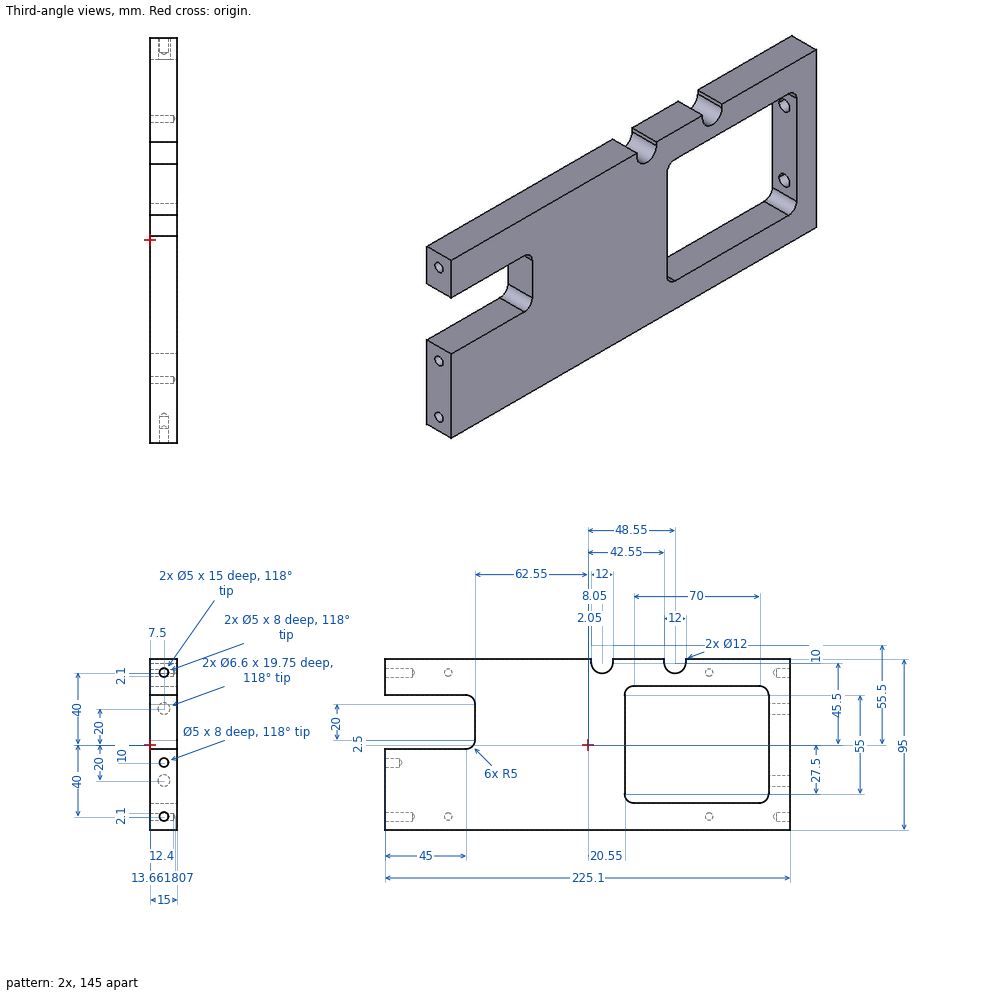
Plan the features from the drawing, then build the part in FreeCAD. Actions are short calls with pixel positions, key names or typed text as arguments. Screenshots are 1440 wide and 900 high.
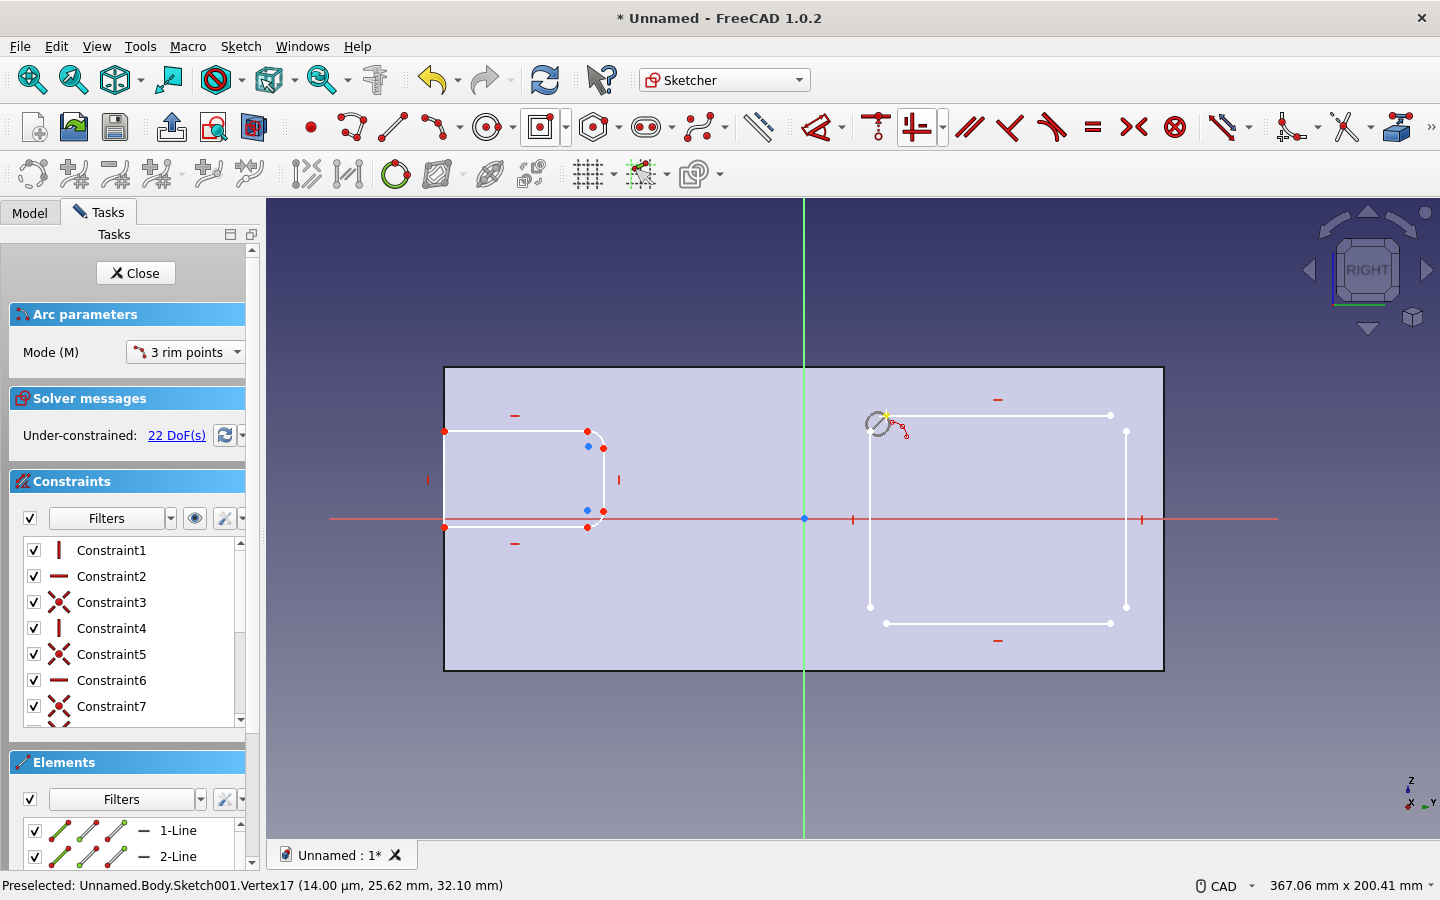
scroll(874, 419, up, 7)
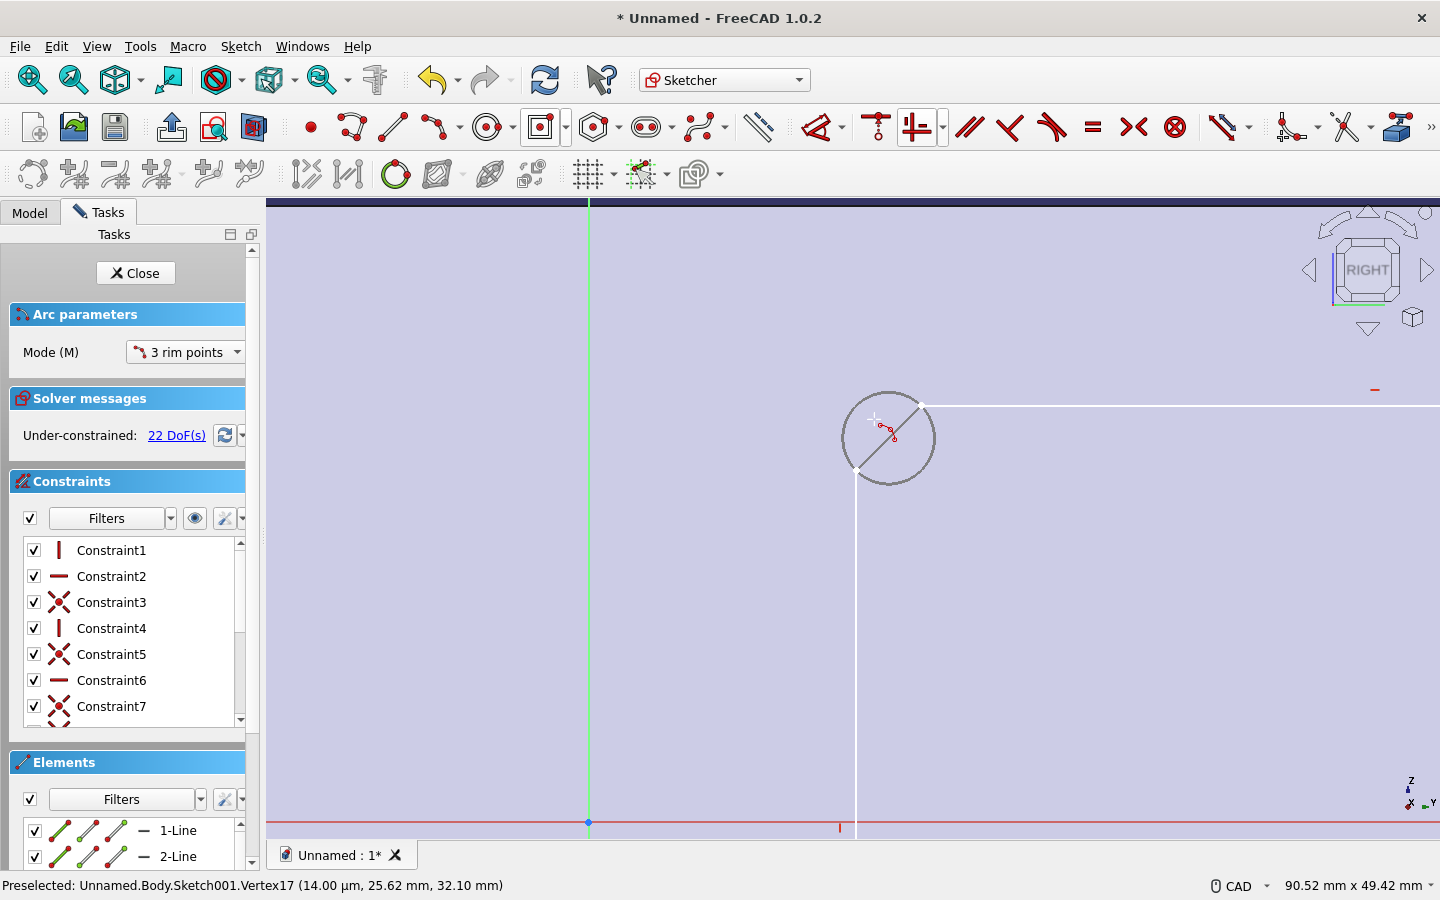
click(874, 420)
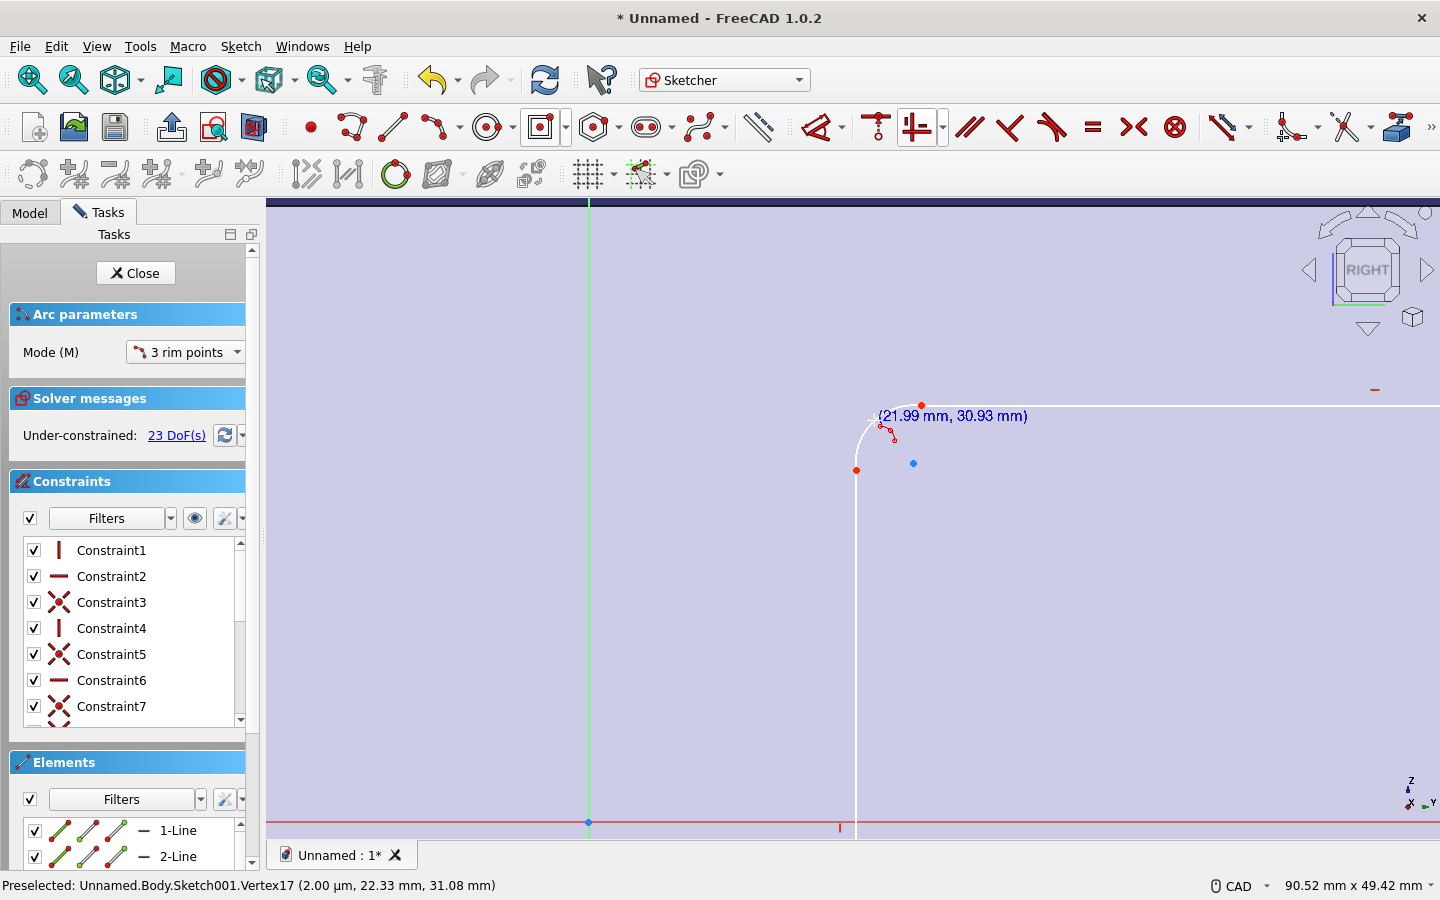
scroll(874, 419, down, 7)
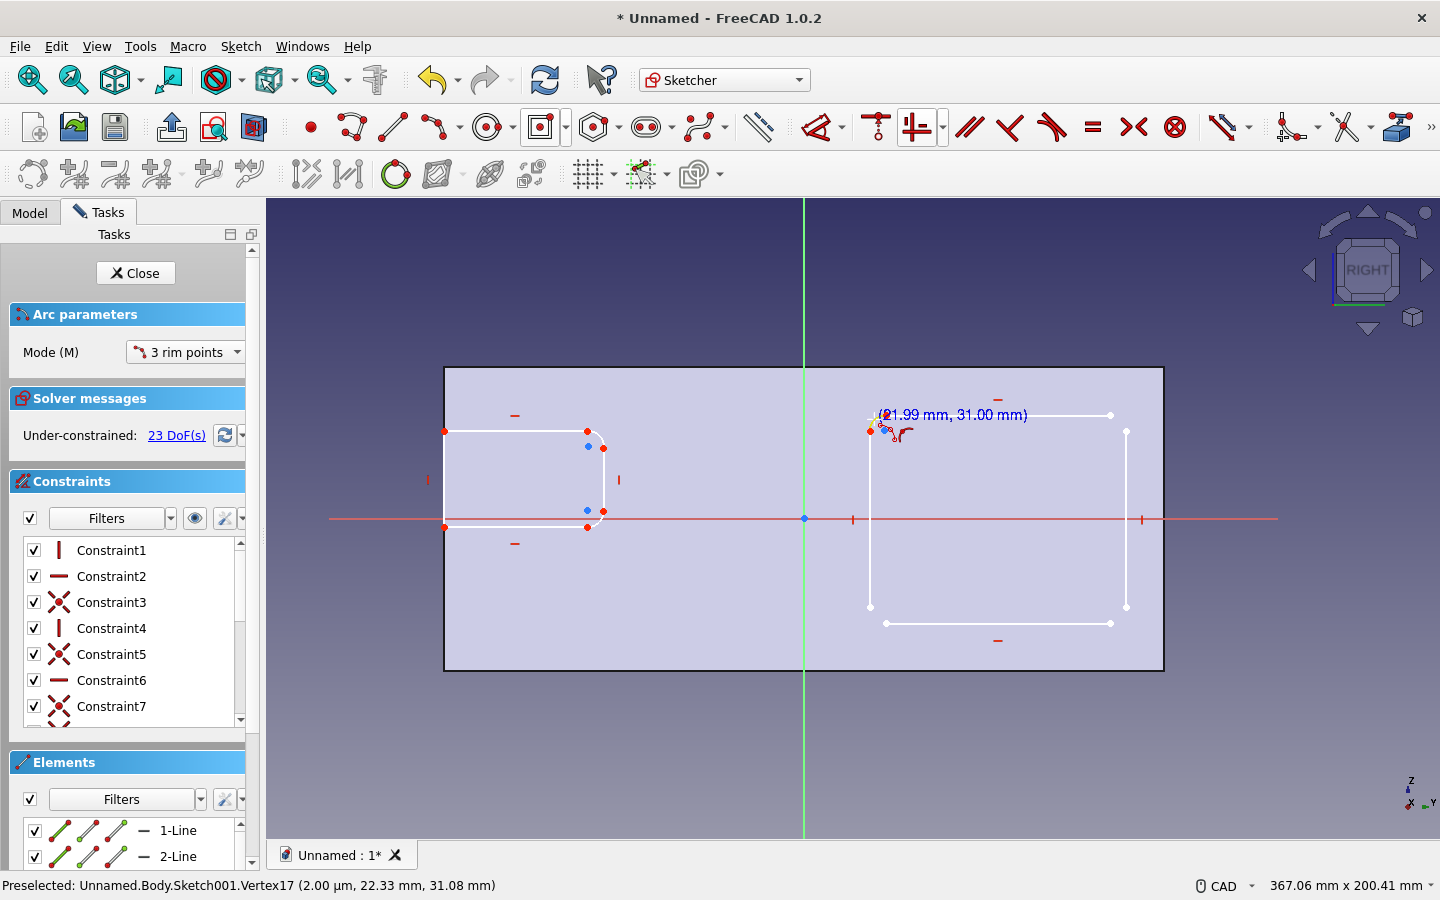
click(1110, 416)
click(1126, 432)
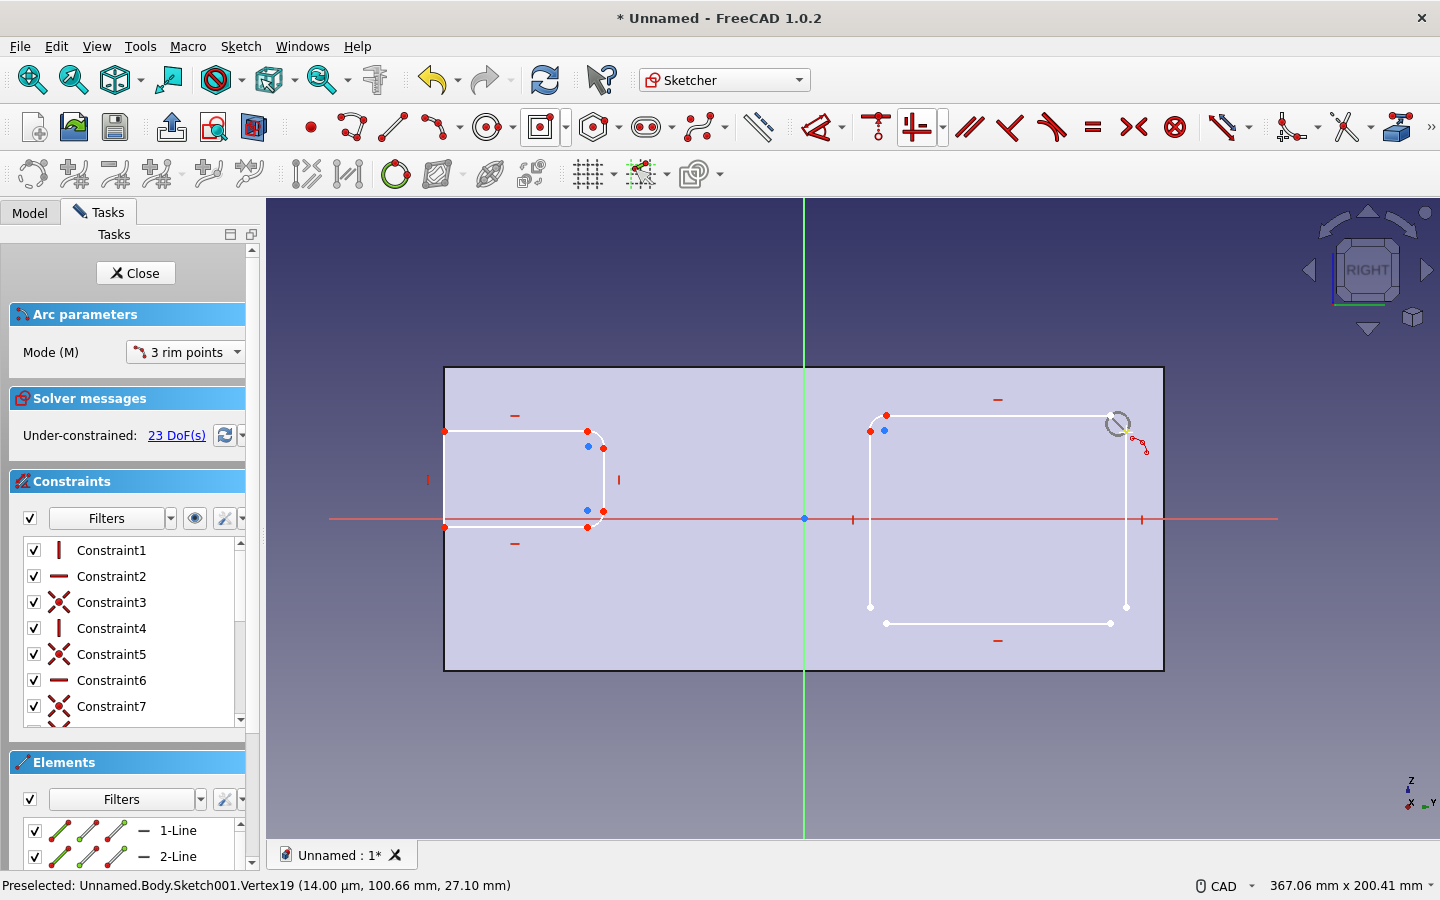
scroll(1121, 419, up, 7)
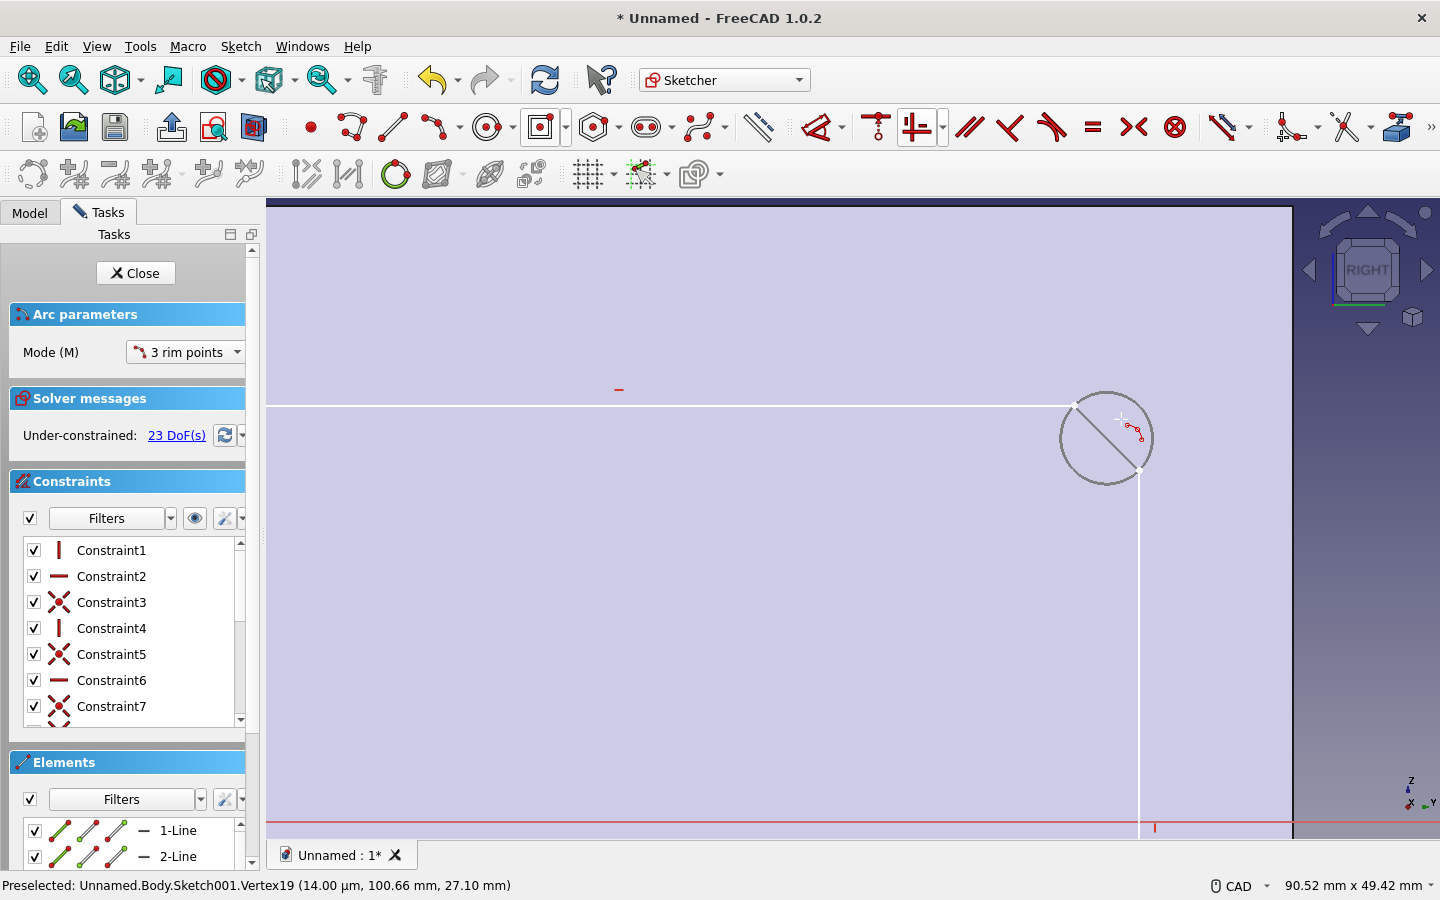
click(1119, 420)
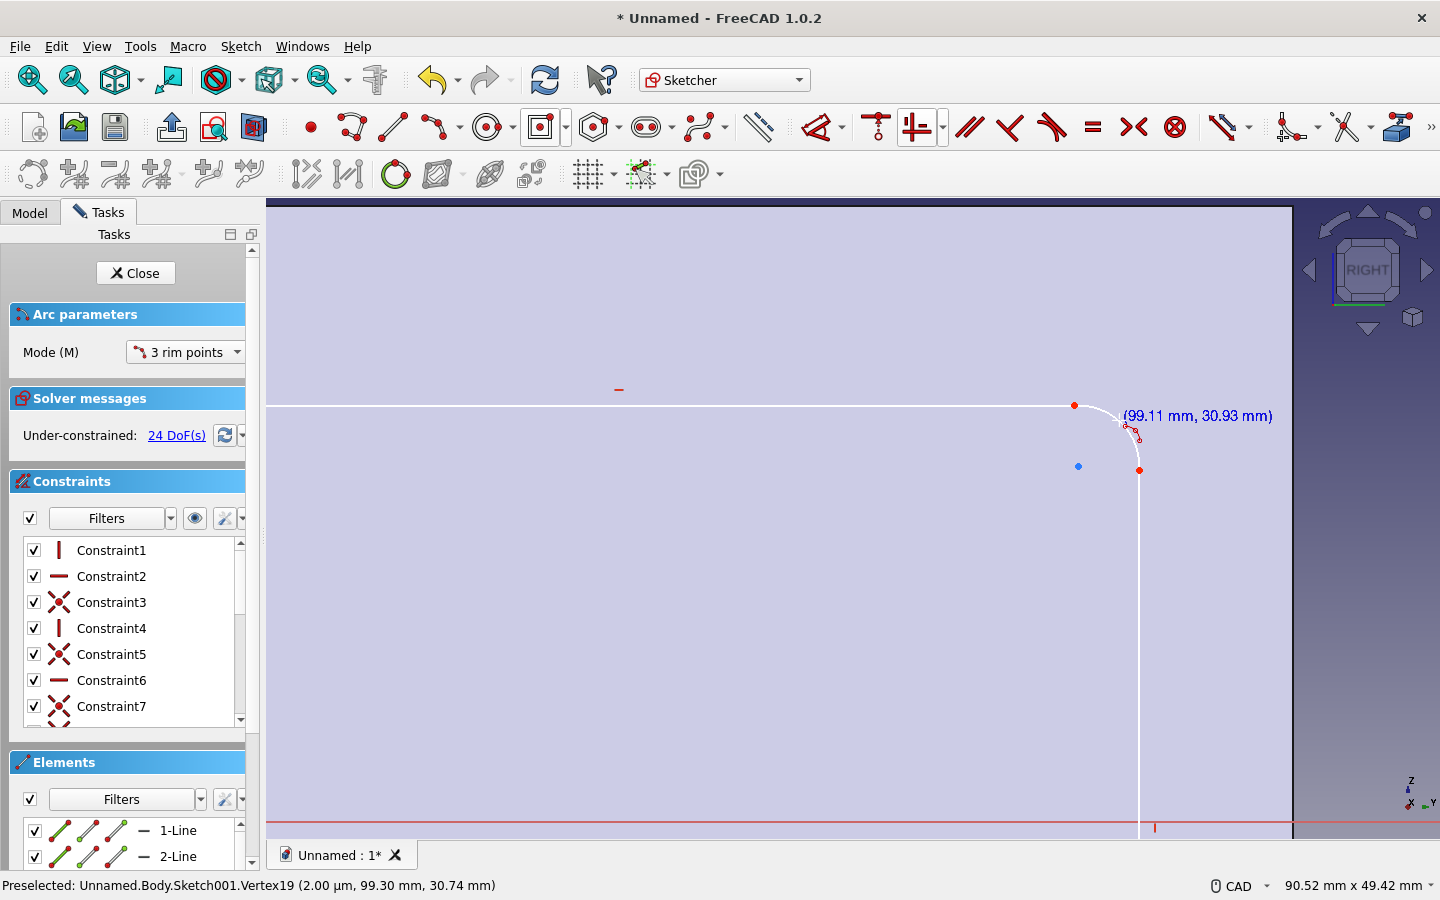
scroll(1121, 419, down, 7)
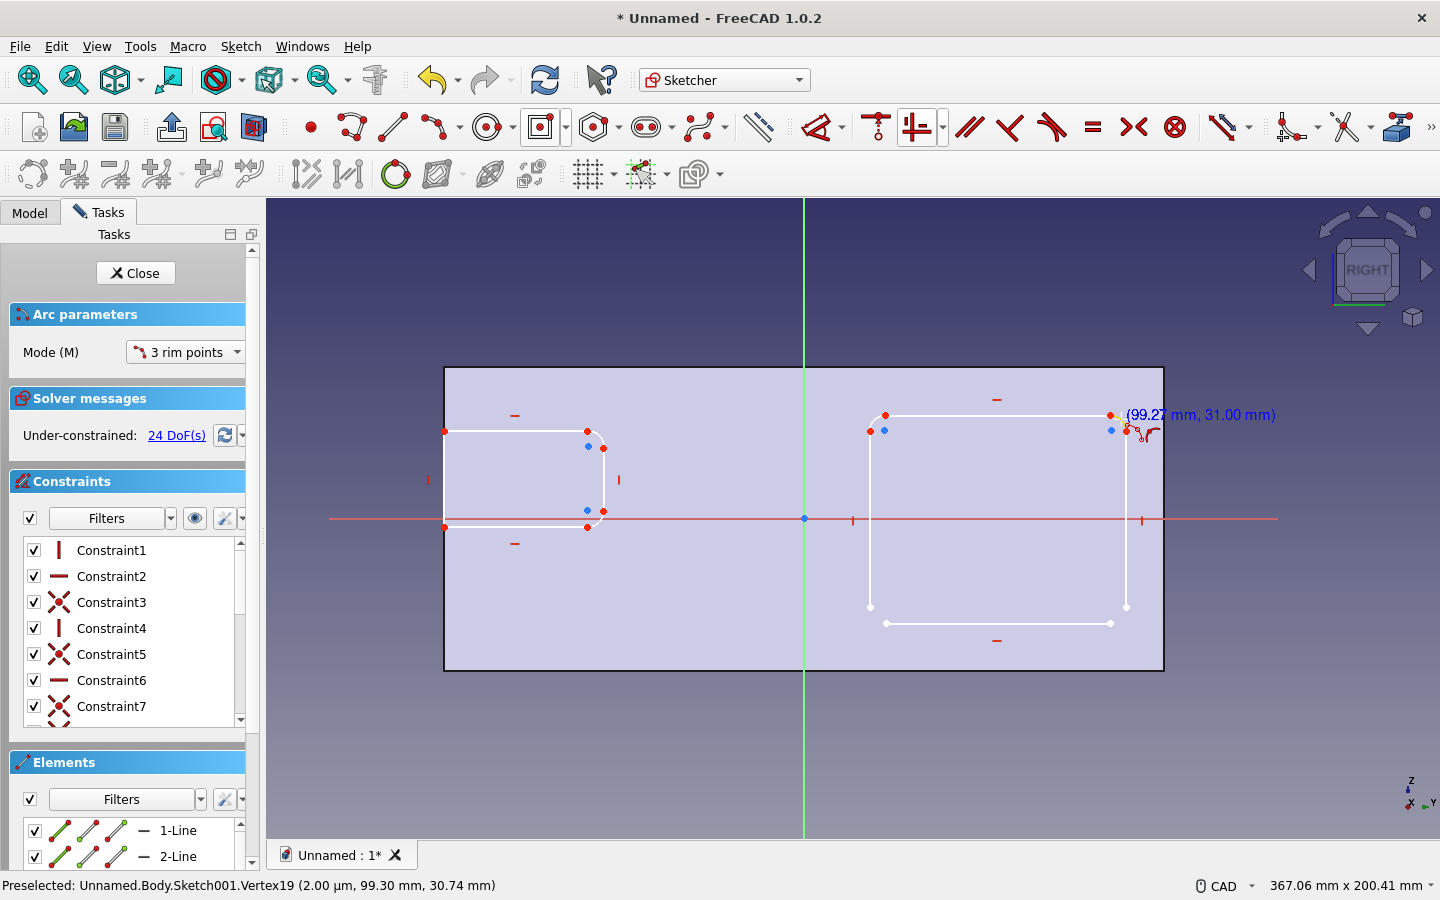
click(1126, 608)
click(1110, 624)